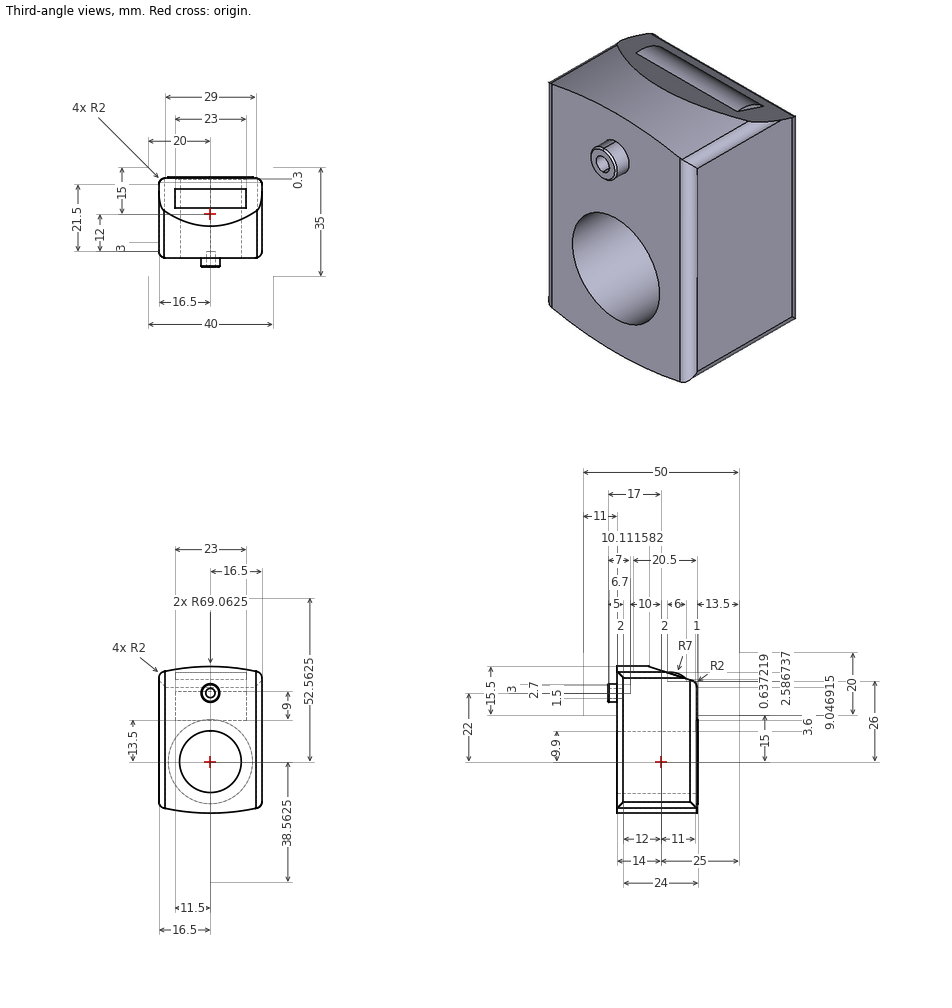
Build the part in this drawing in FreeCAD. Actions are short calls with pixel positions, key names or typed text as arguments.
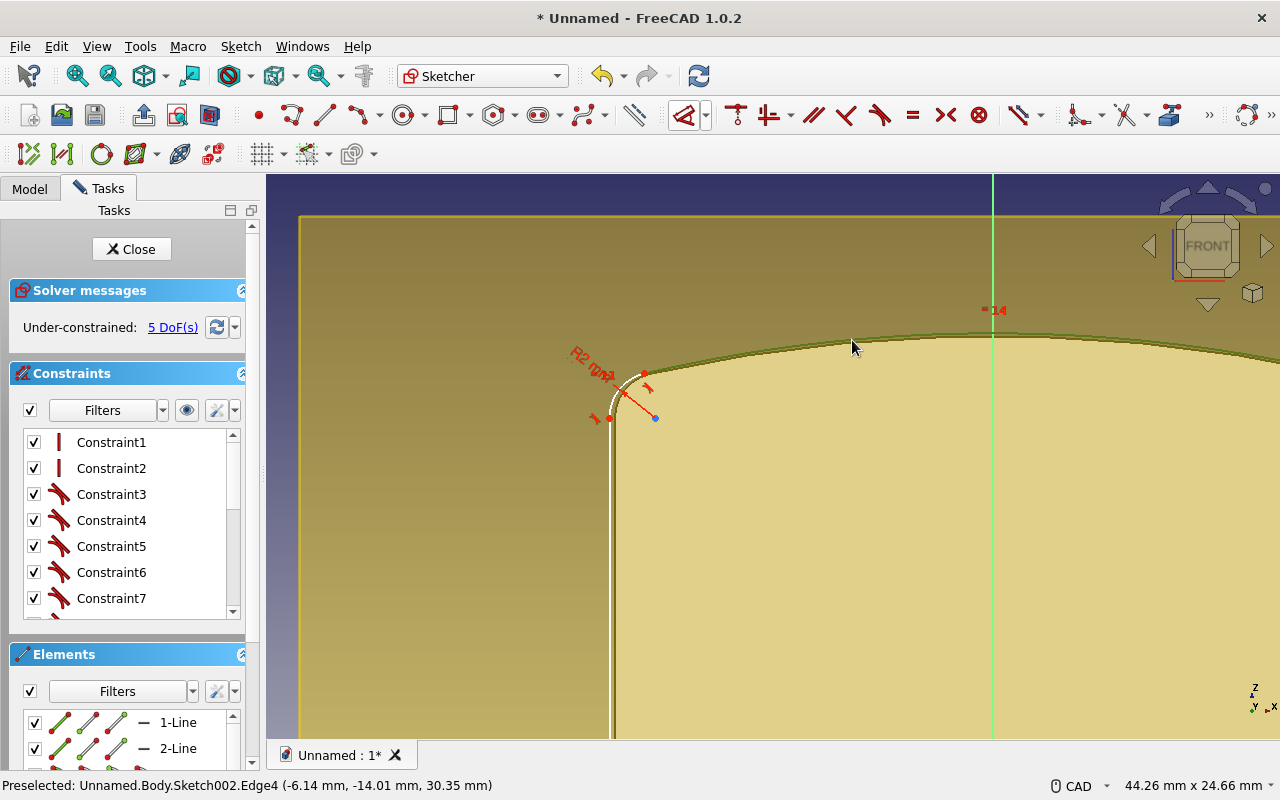
click(706, 116)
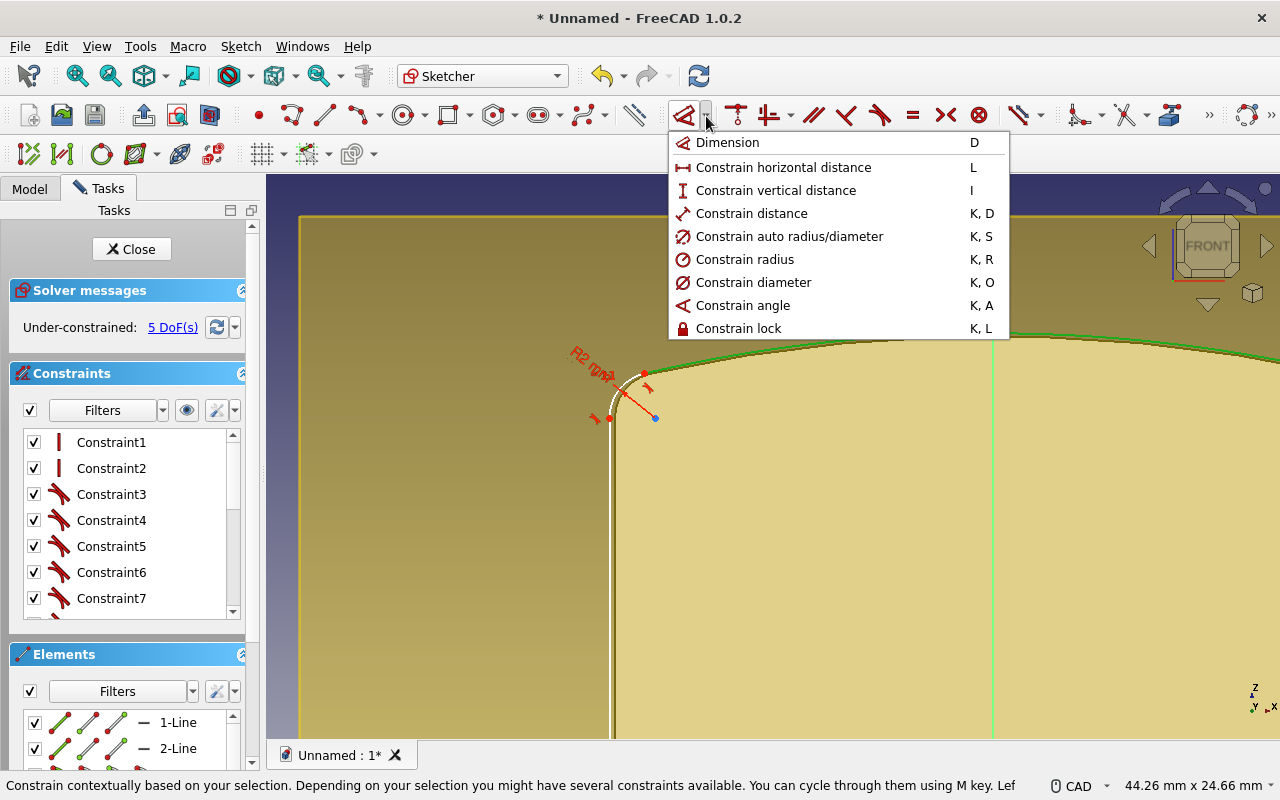
click(839, 260)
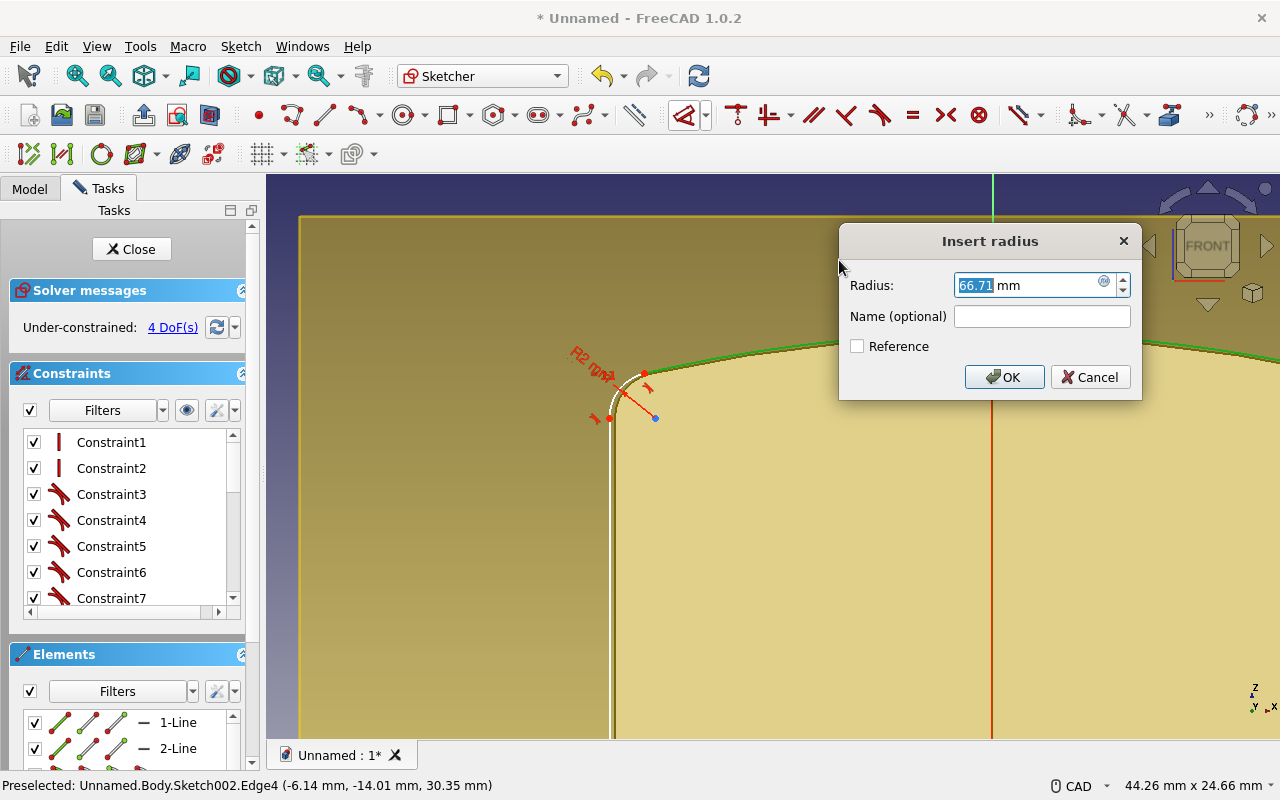
text(69.0625)
key(Return)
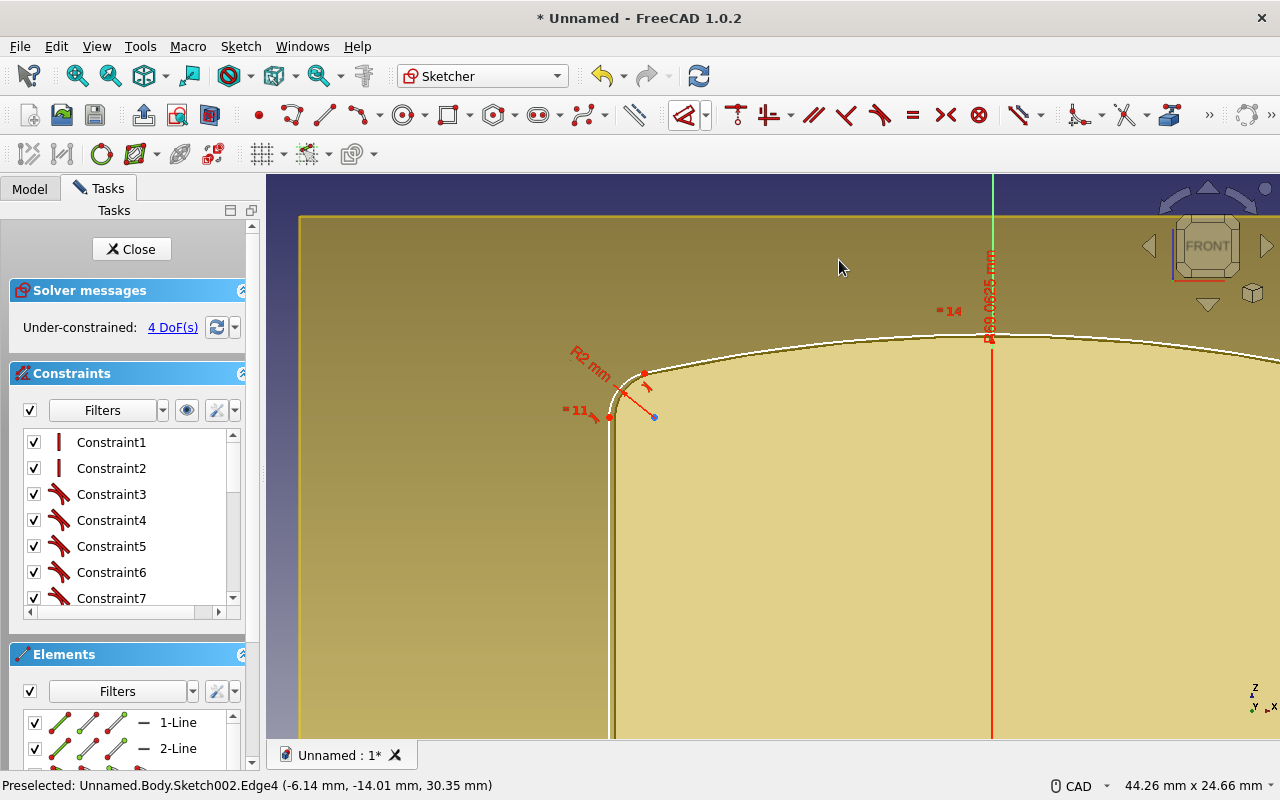
scroll(537, 213, down, 5)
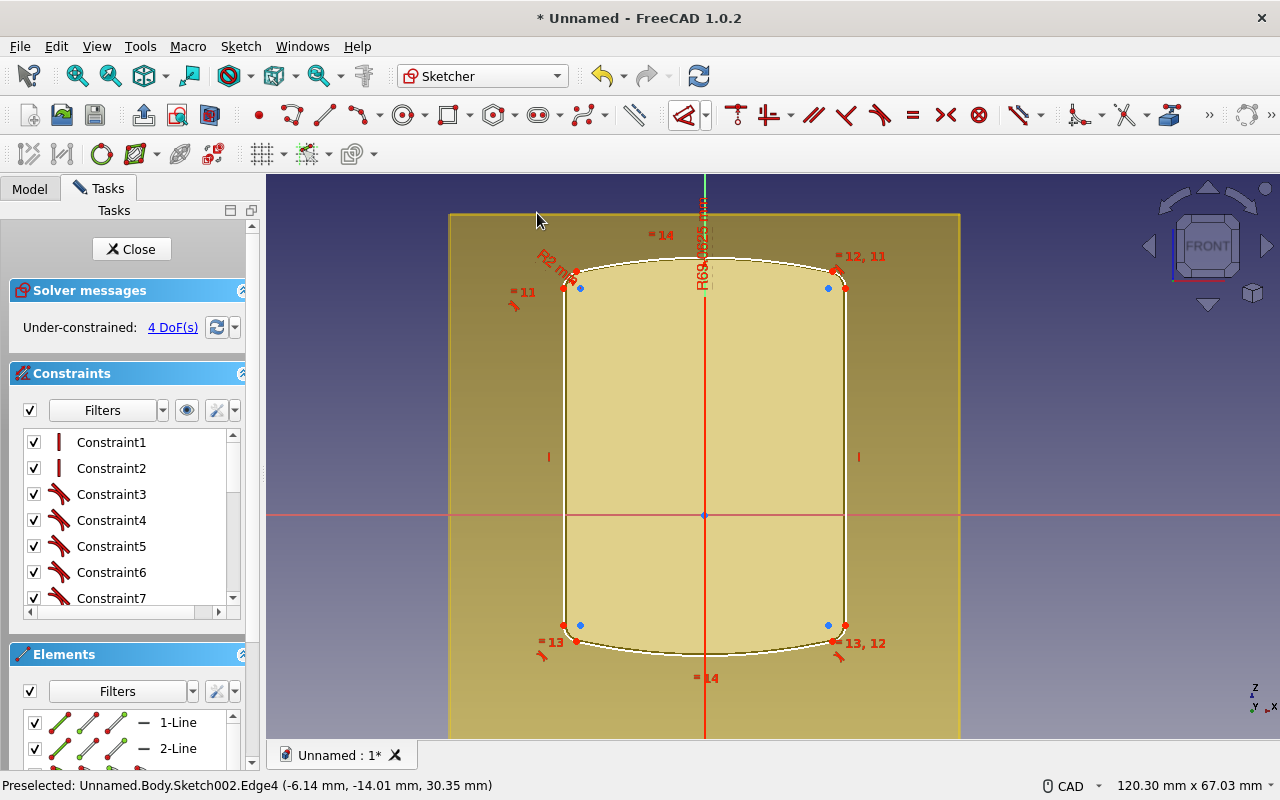
click(564, 625)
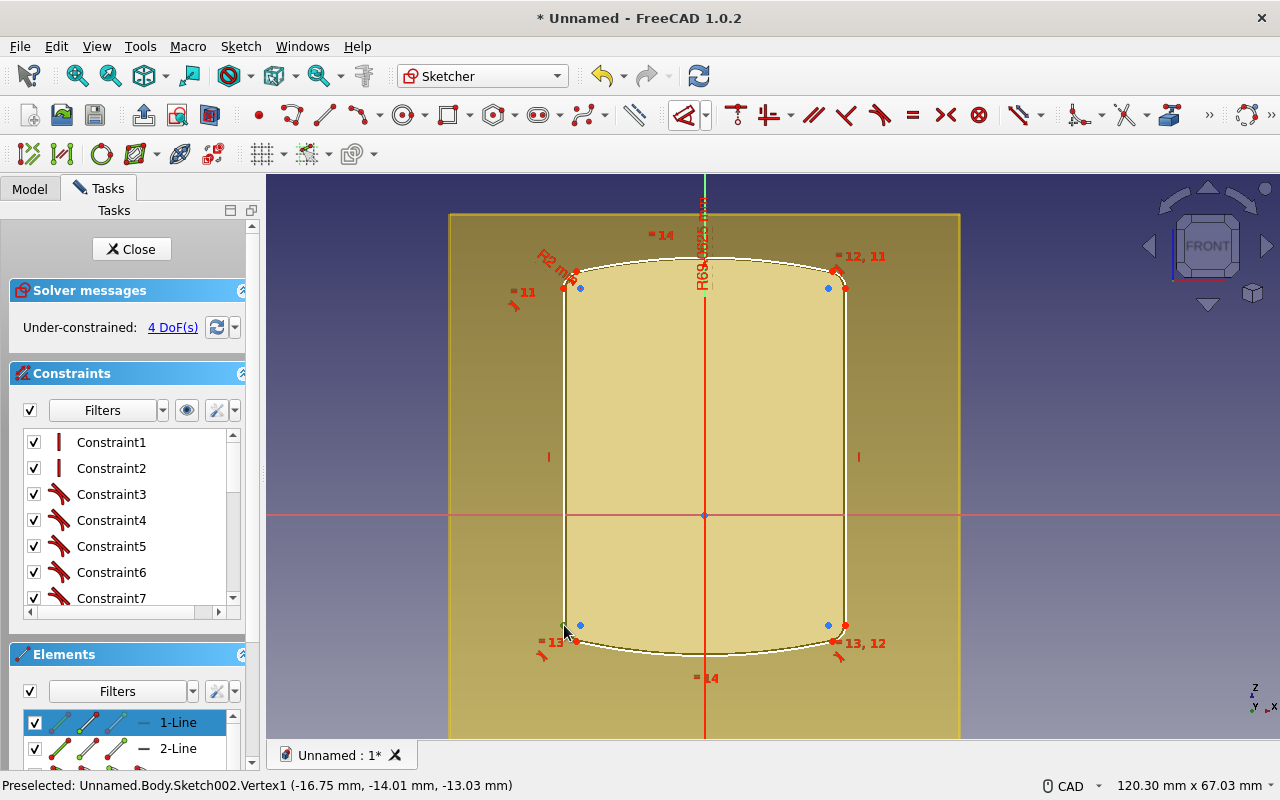
key(l)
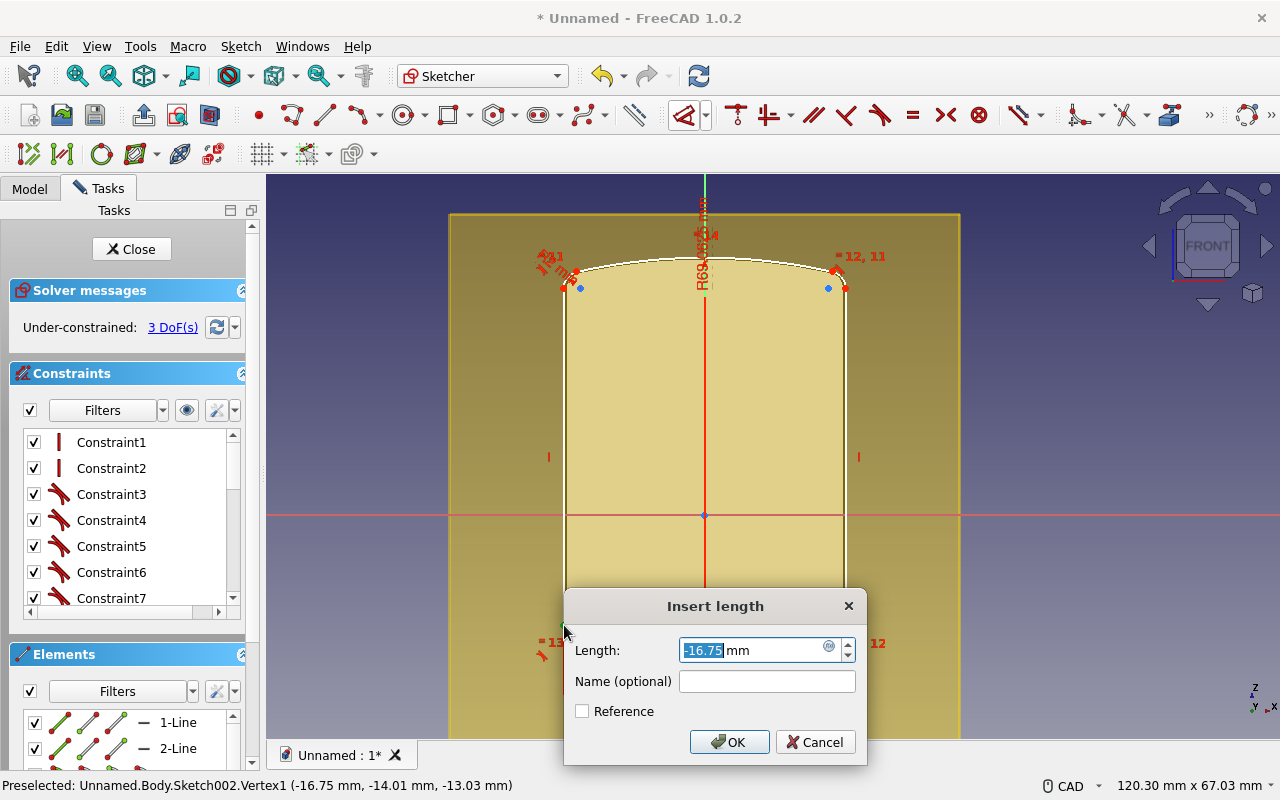
text(-16.5)
key(Return)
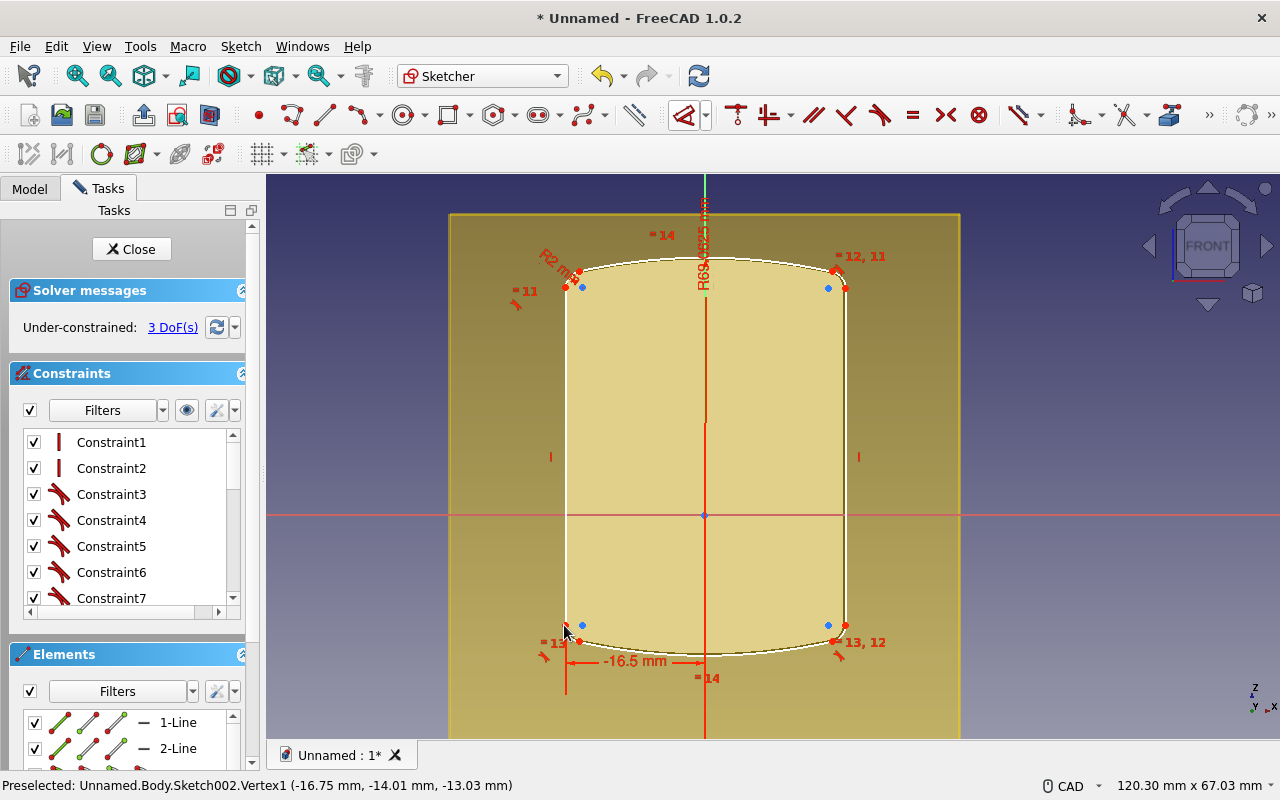
click(846, 288)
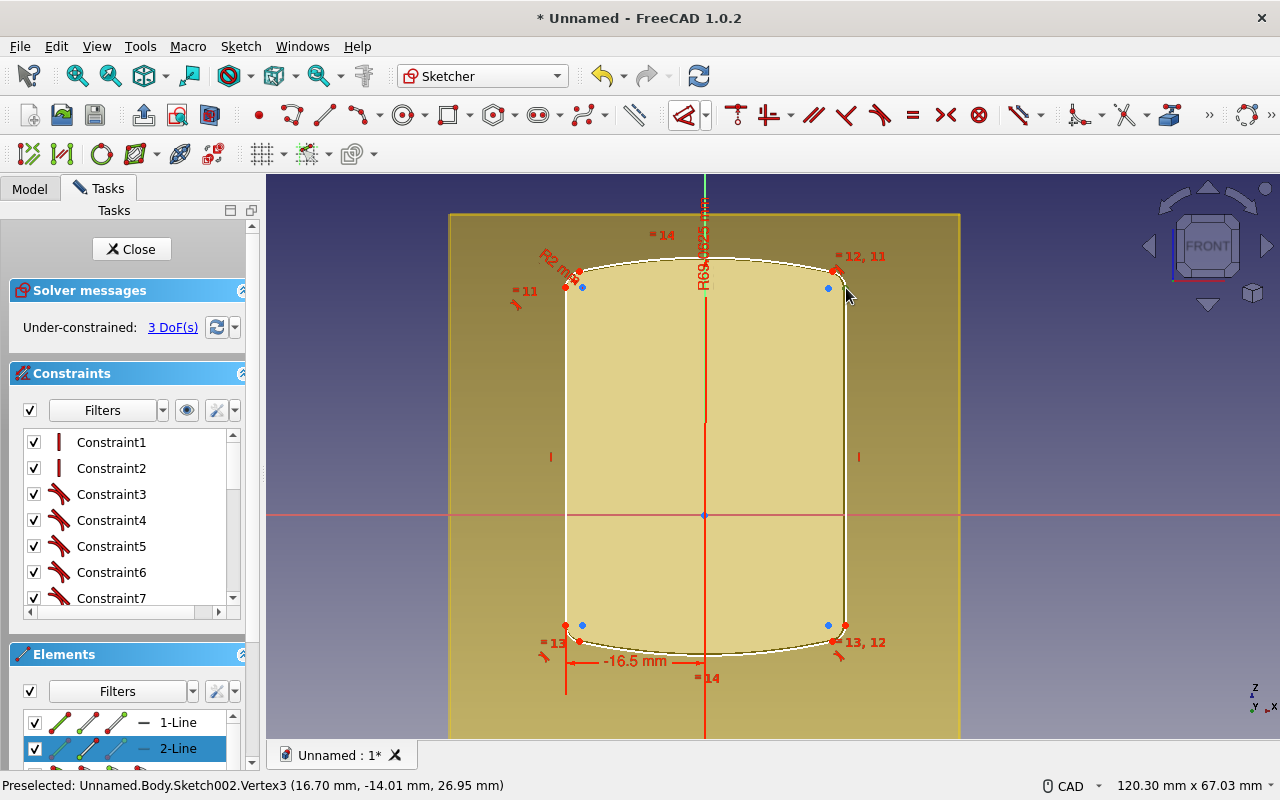
click(706, 116)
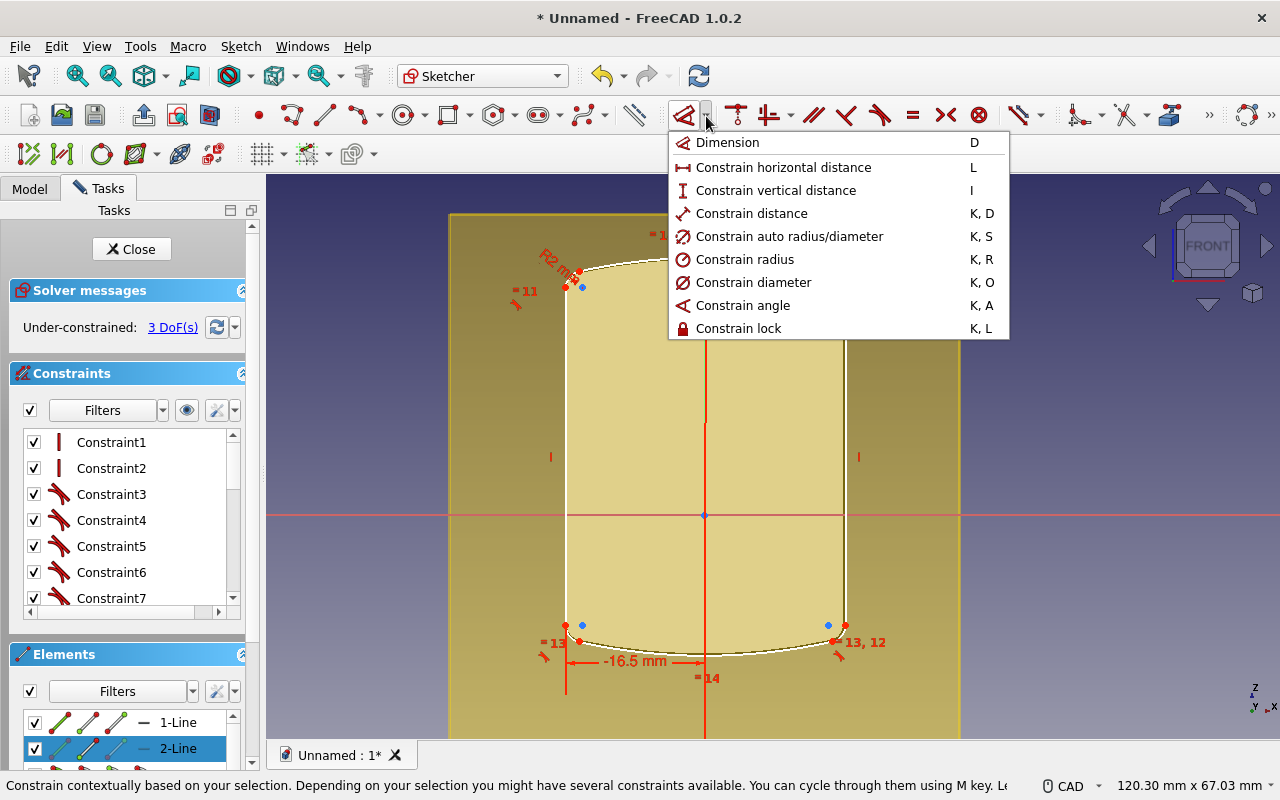
click(839, 168)